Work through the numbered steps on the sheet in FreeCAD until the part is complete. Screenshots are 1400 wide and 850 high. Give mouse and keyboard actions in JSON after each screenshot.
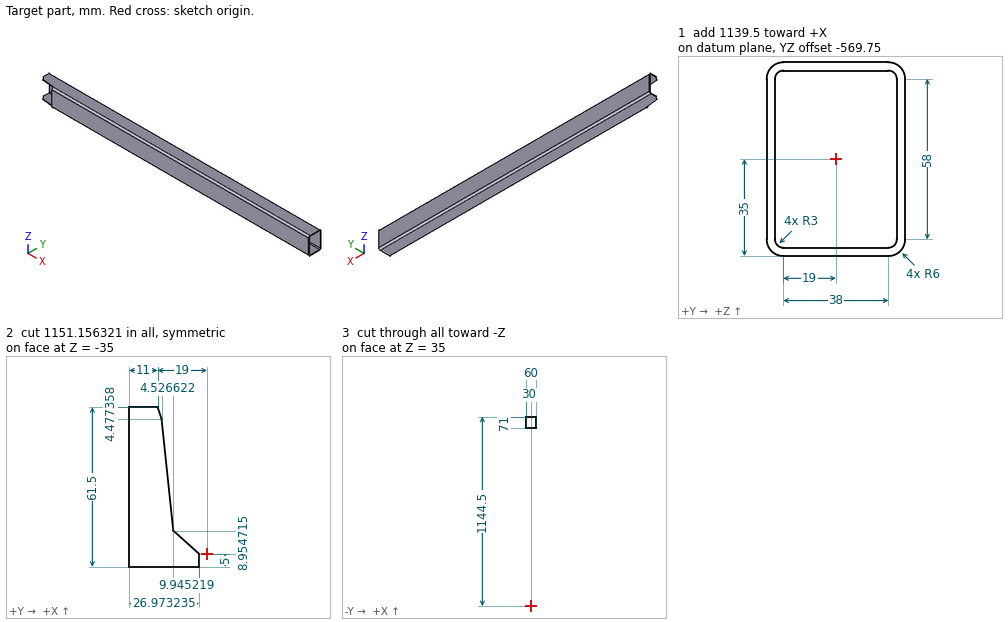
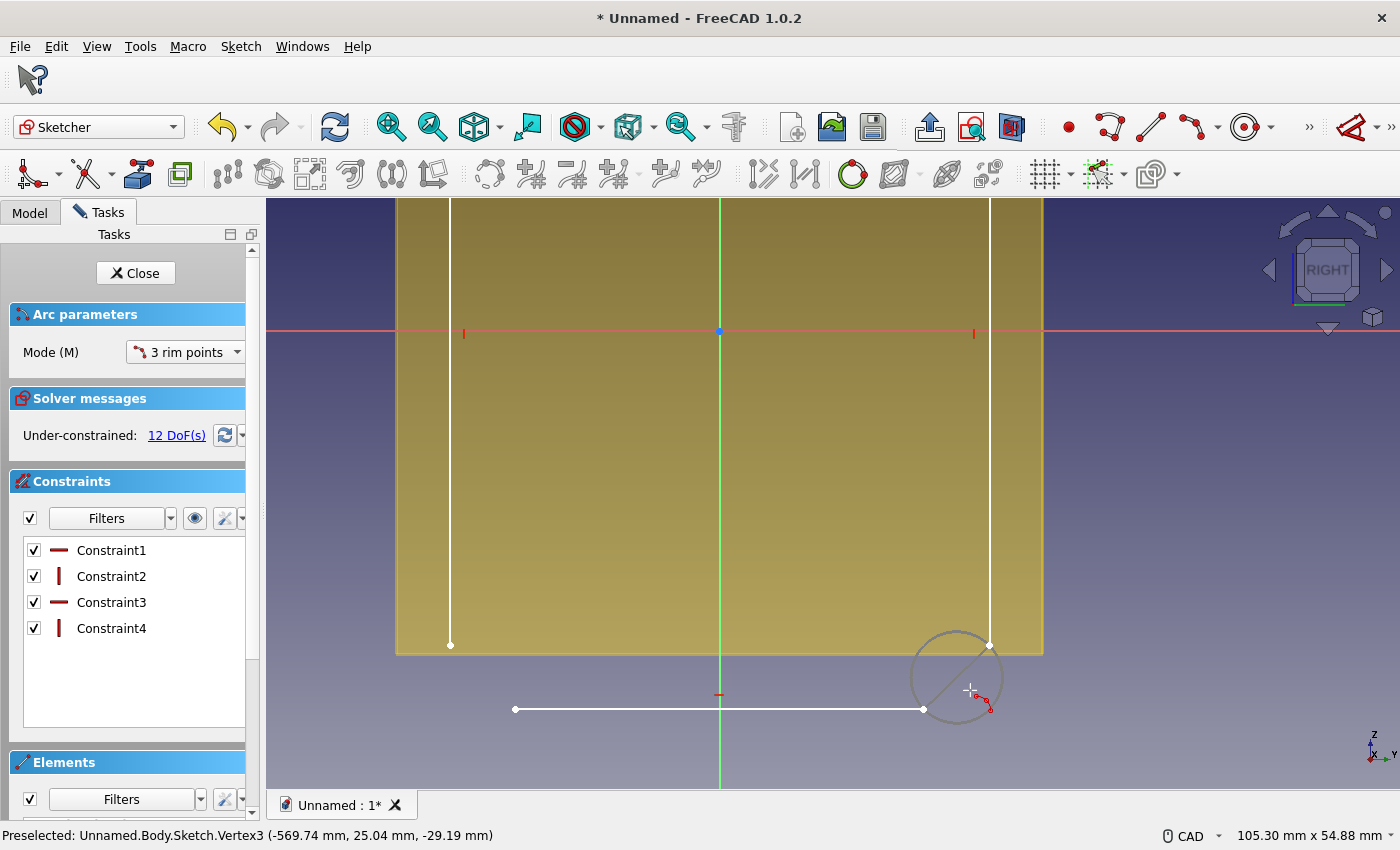
{"action": "left_click", "coordinate": [970, 689]}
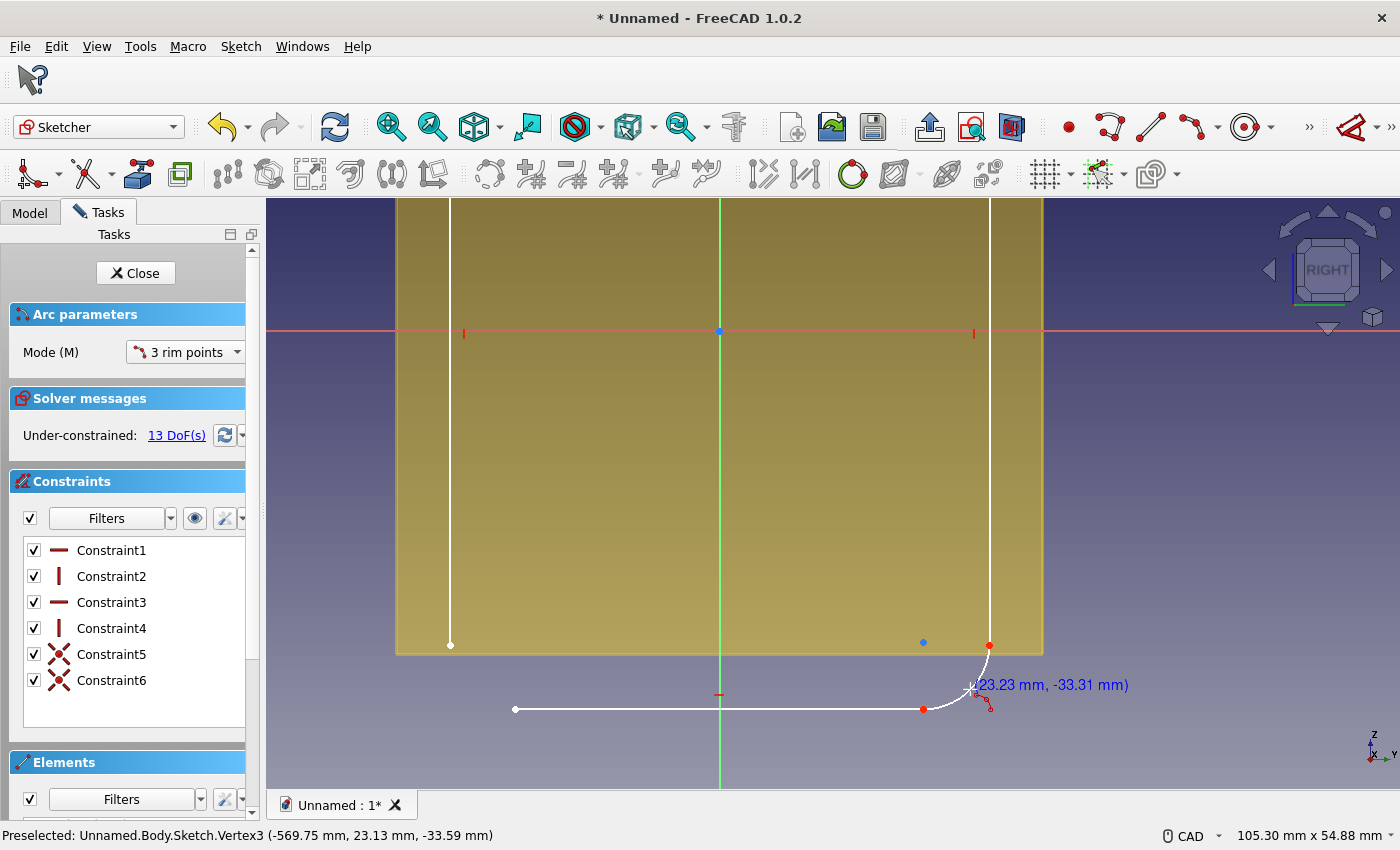
{"action": "scroll", "coordinate": [819, 691], "scroll_direction": "down", "scroll_amount": 3}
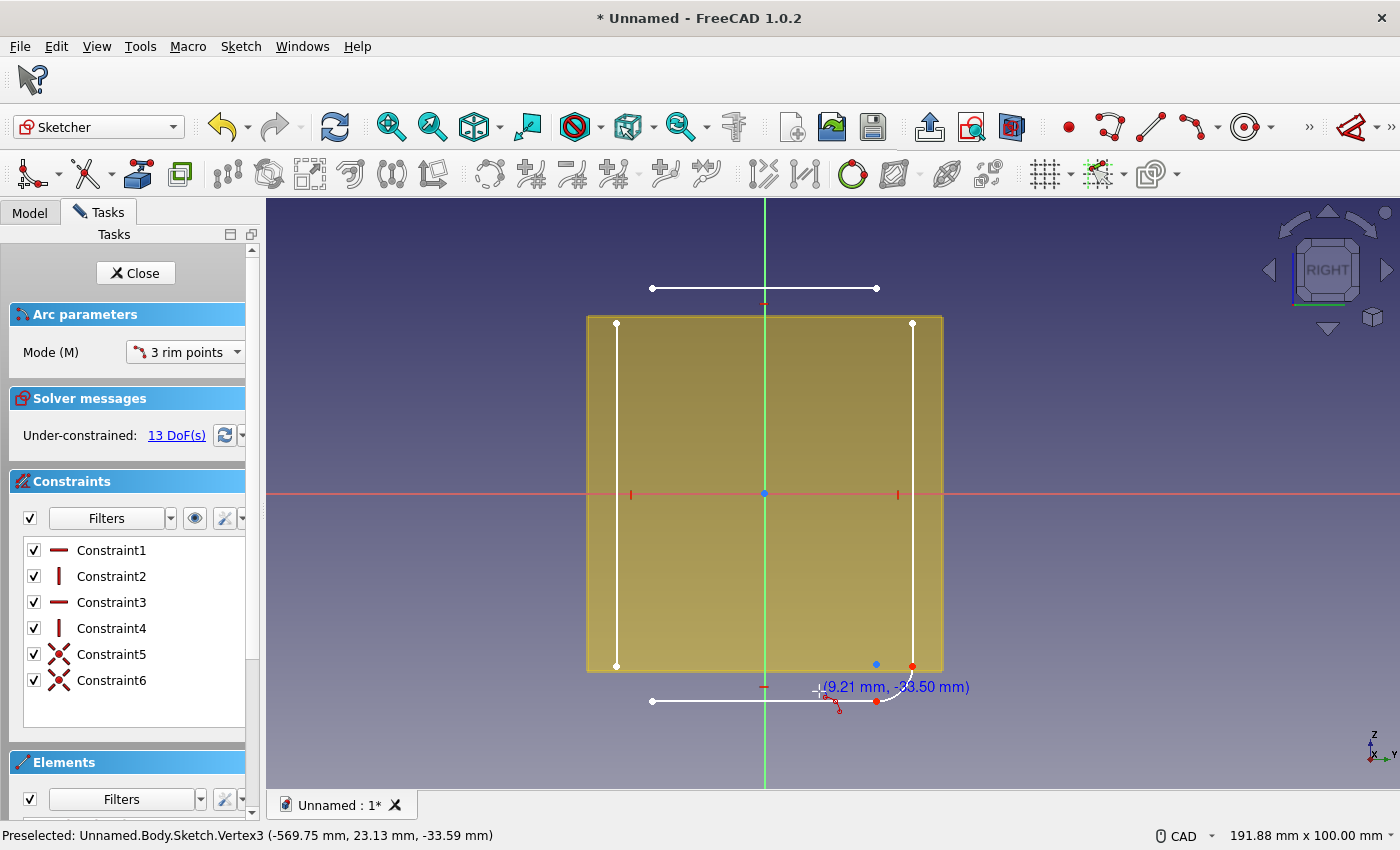
{"action": "left_click", "coordinate": [913, 323]}
{"action": "left_click", "coordinate": [877, 288]}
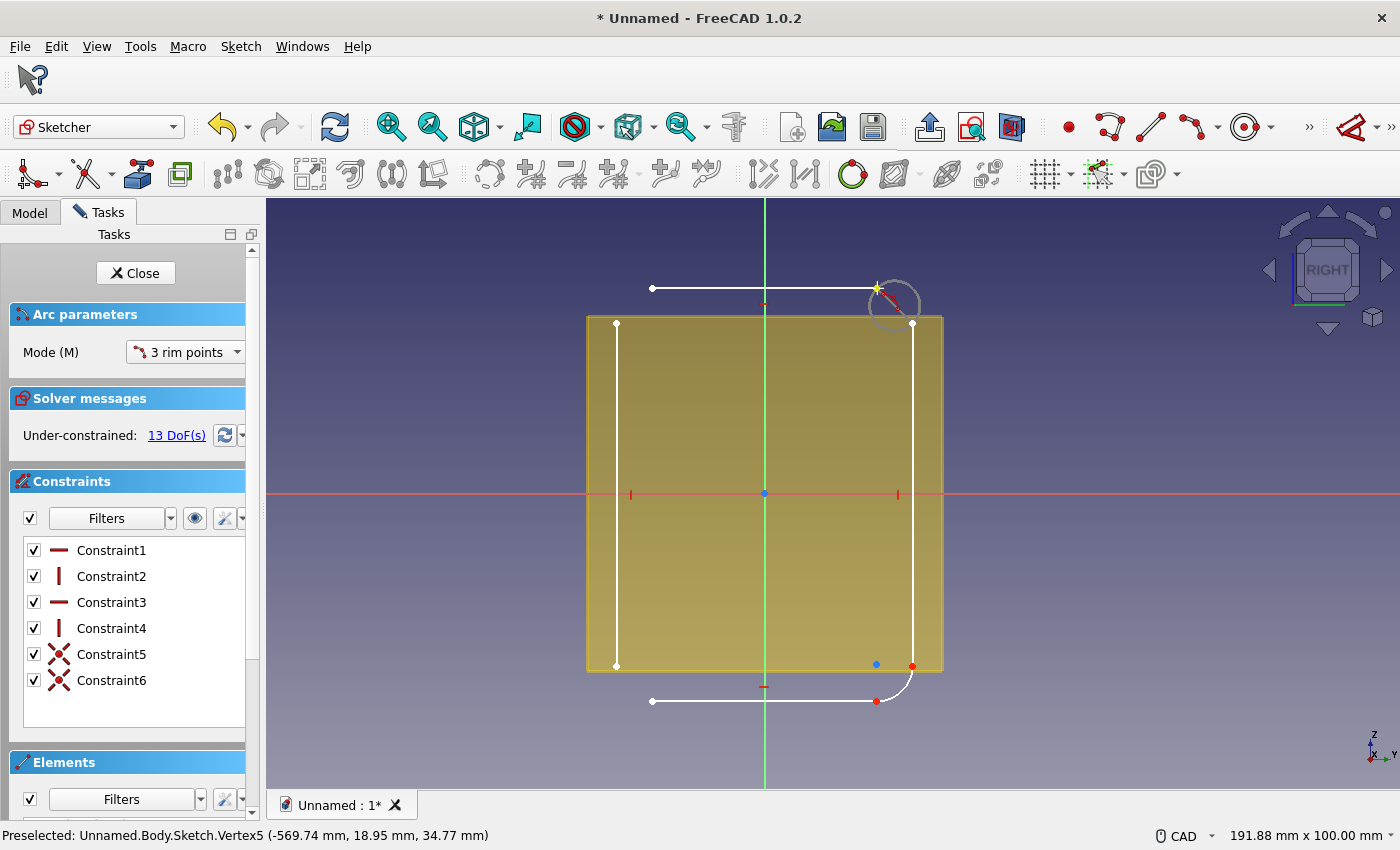
{"action": "scroll", "coordinate": [902, 297], "scroll_direction": "up", "scroll_amount": 3}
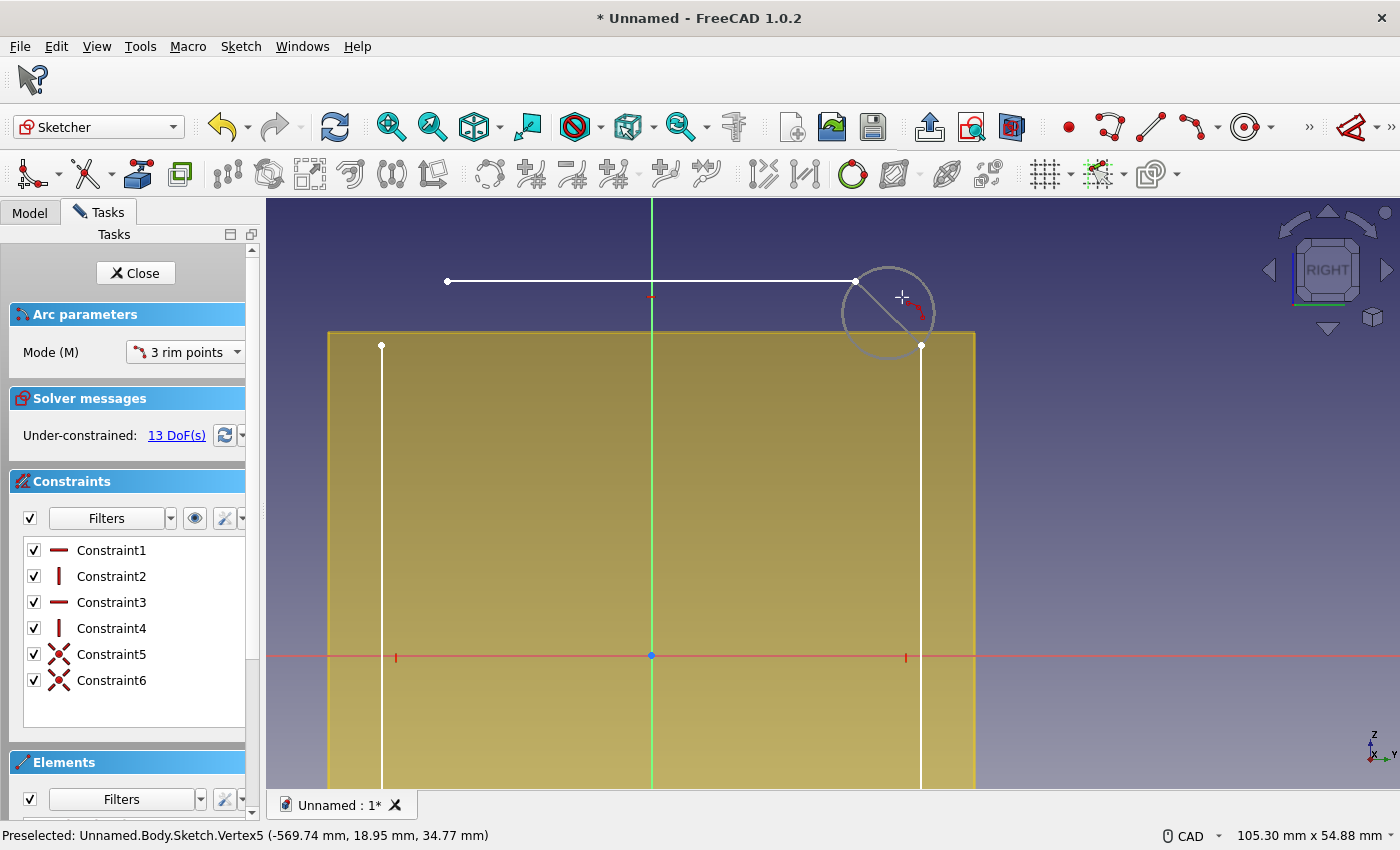
{"action": "left_click", "coordinate": [902, 298]}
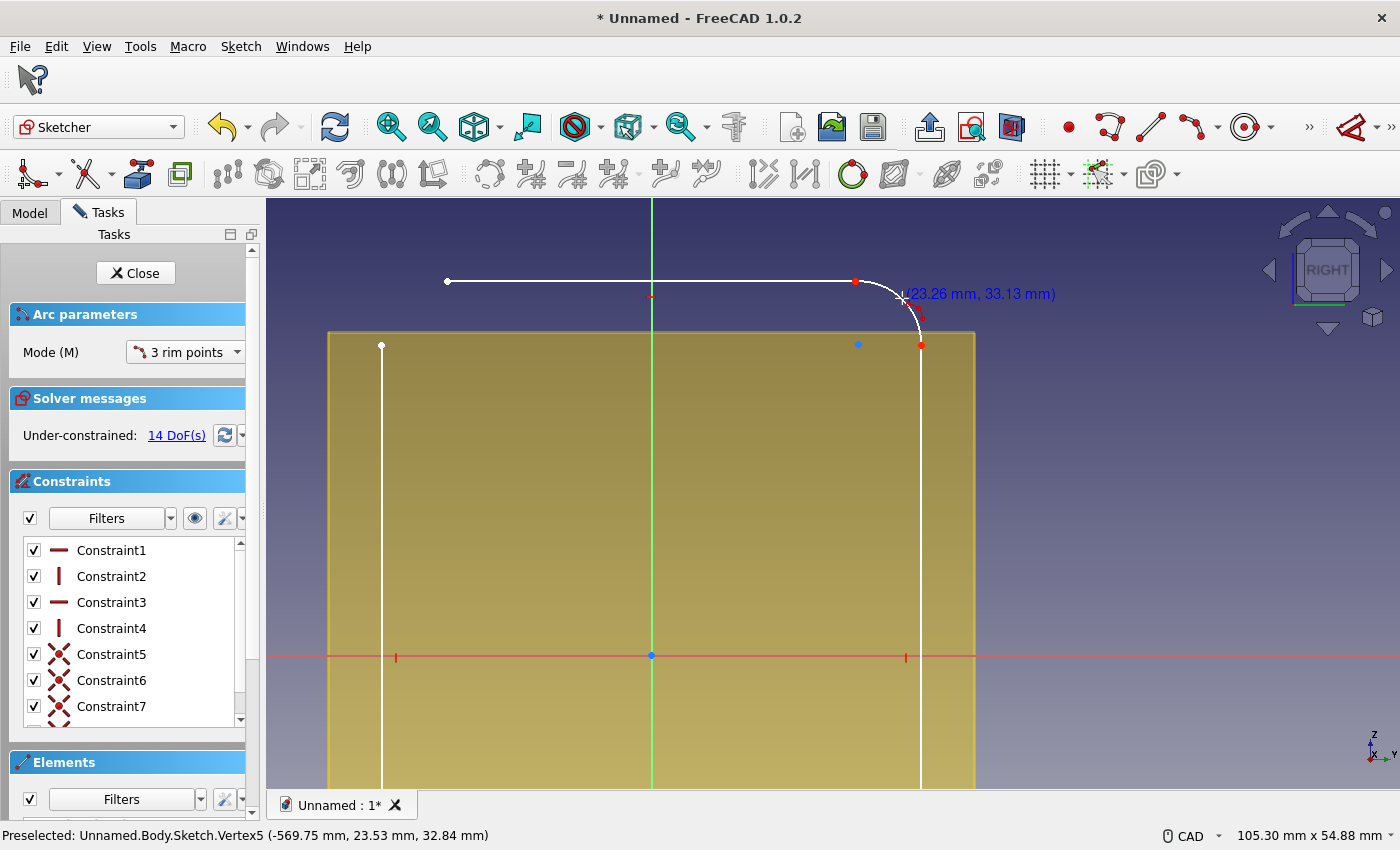
{"action": "left_click", "coordinate": [447, 281]}
{"action": "left_click", "coordinate": [382, 345]}
{"action": "left_click", "coordinate": [401, 298]}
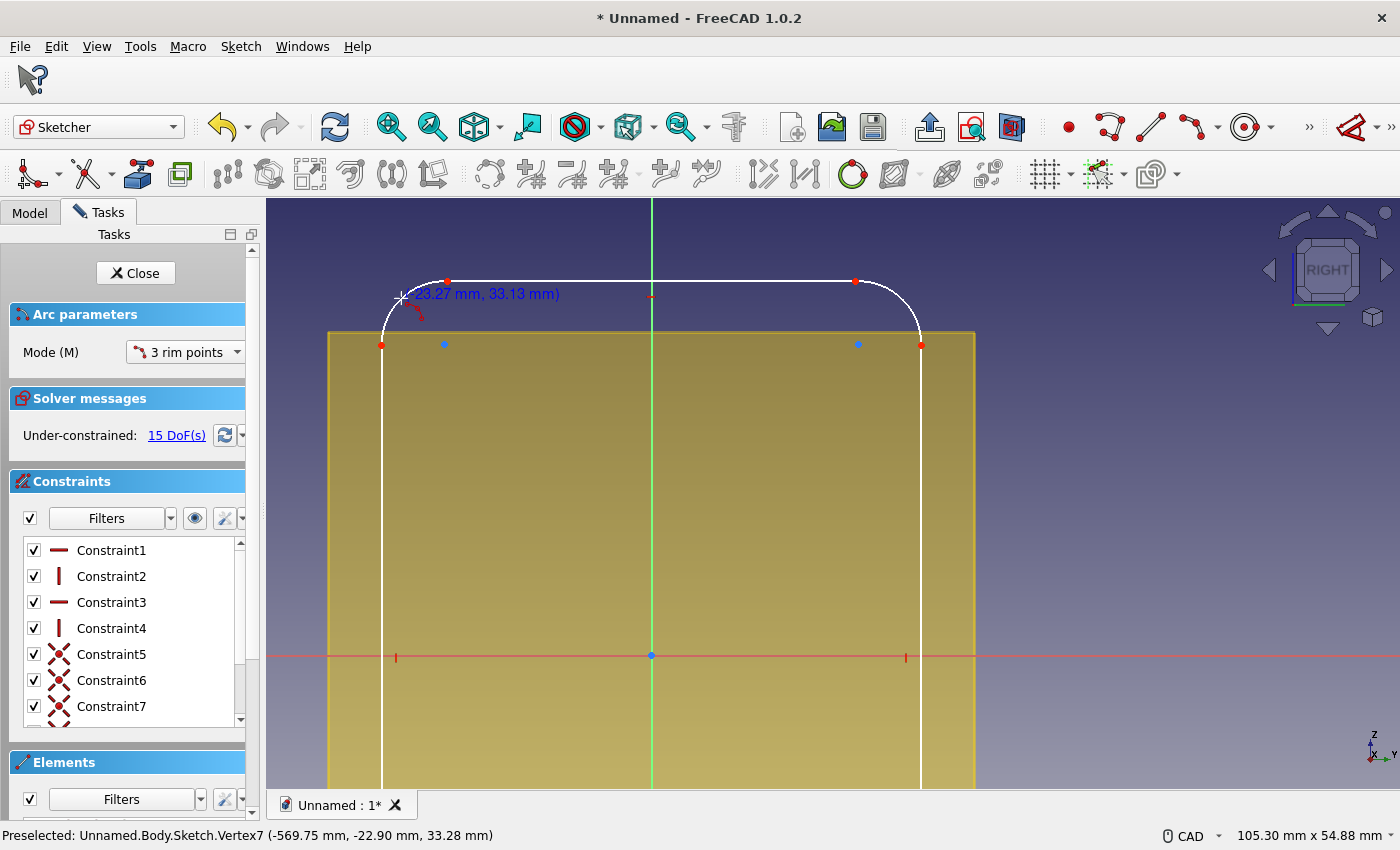
{"action": "scroll", "coordinate": [902, 296], "scroll_direction": "down", "scroll_amount": 3}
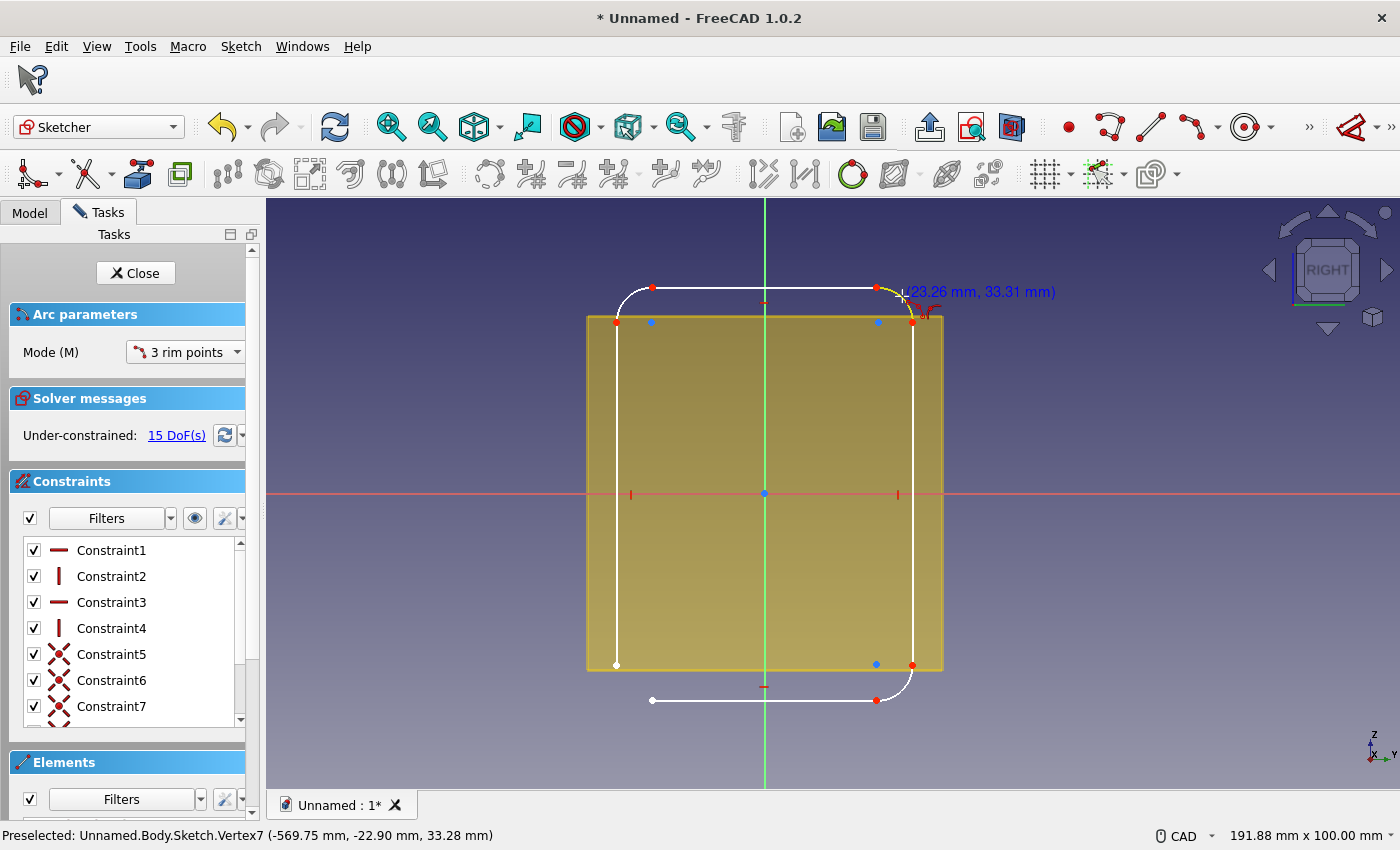
{"action": "left_click", "coordinate": [617, 666]}
{"action": "left_click", "coordinate": [653, 701]}